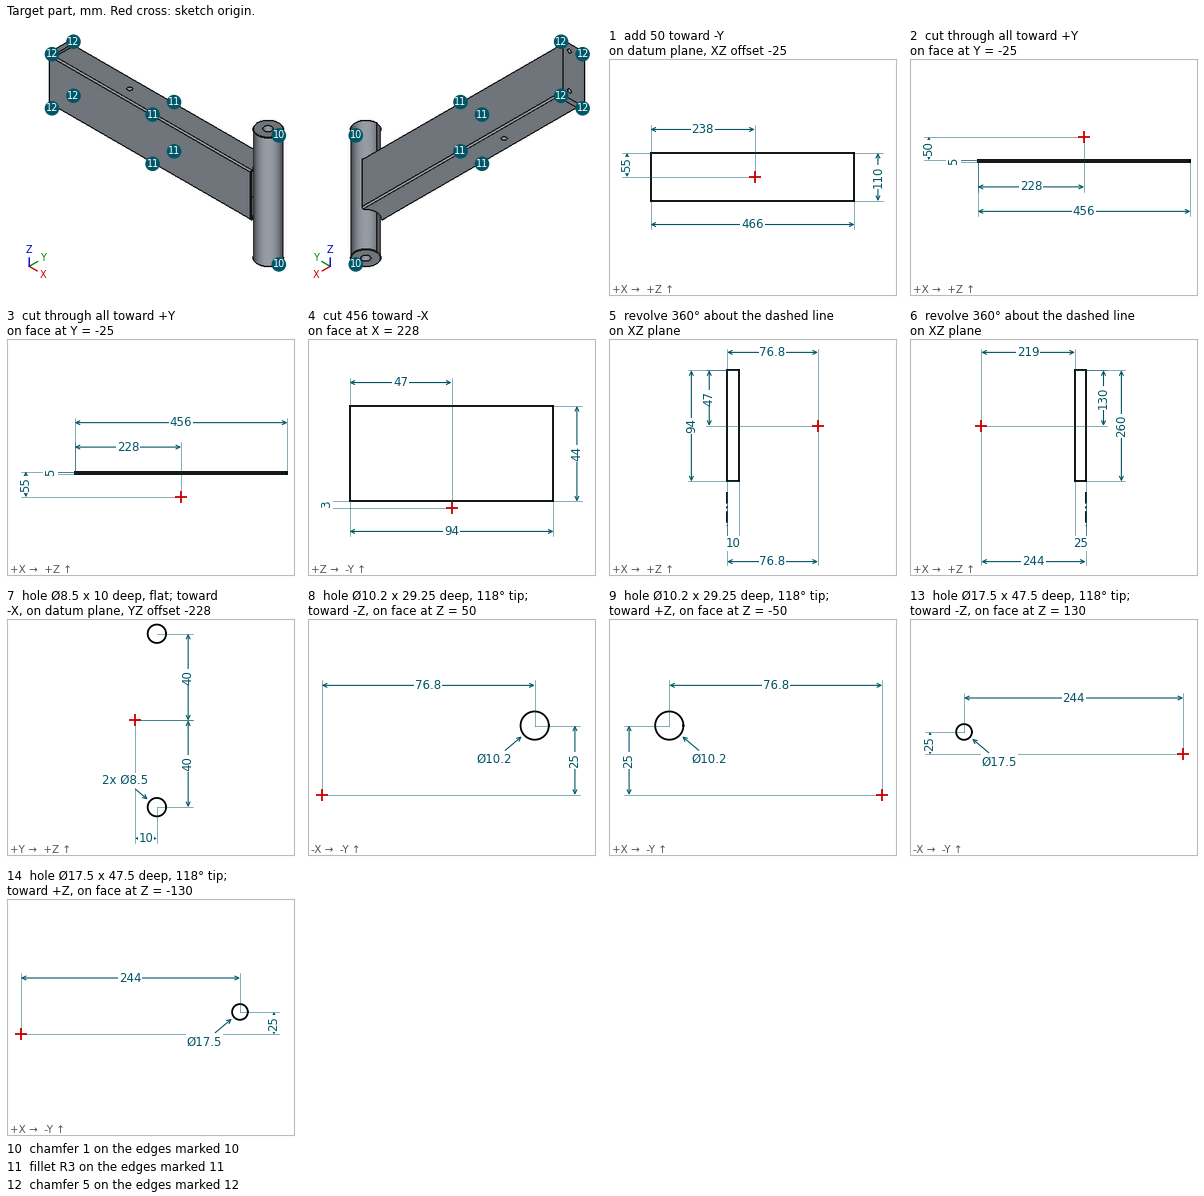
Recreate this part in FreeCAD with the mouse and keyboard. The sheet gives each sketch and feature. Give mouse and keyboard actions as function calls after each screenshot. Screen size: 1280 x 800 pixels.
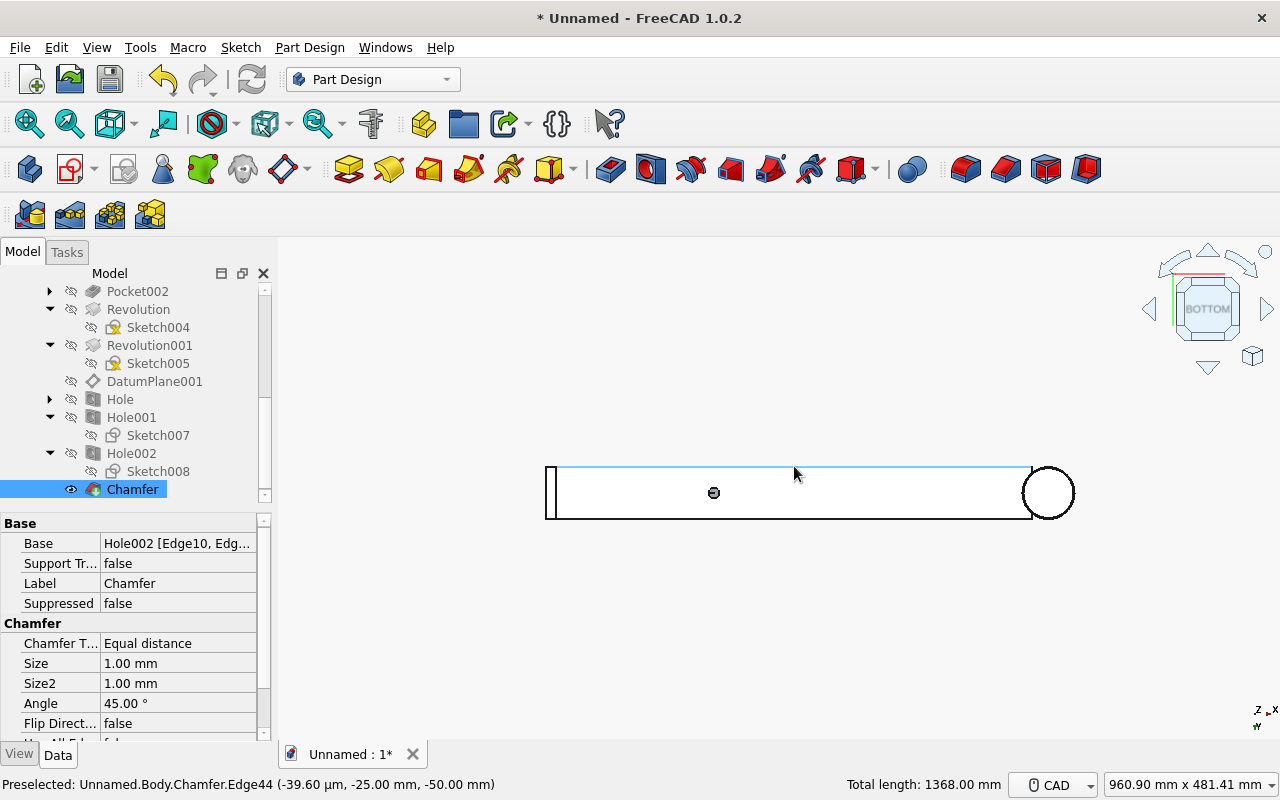
key(4)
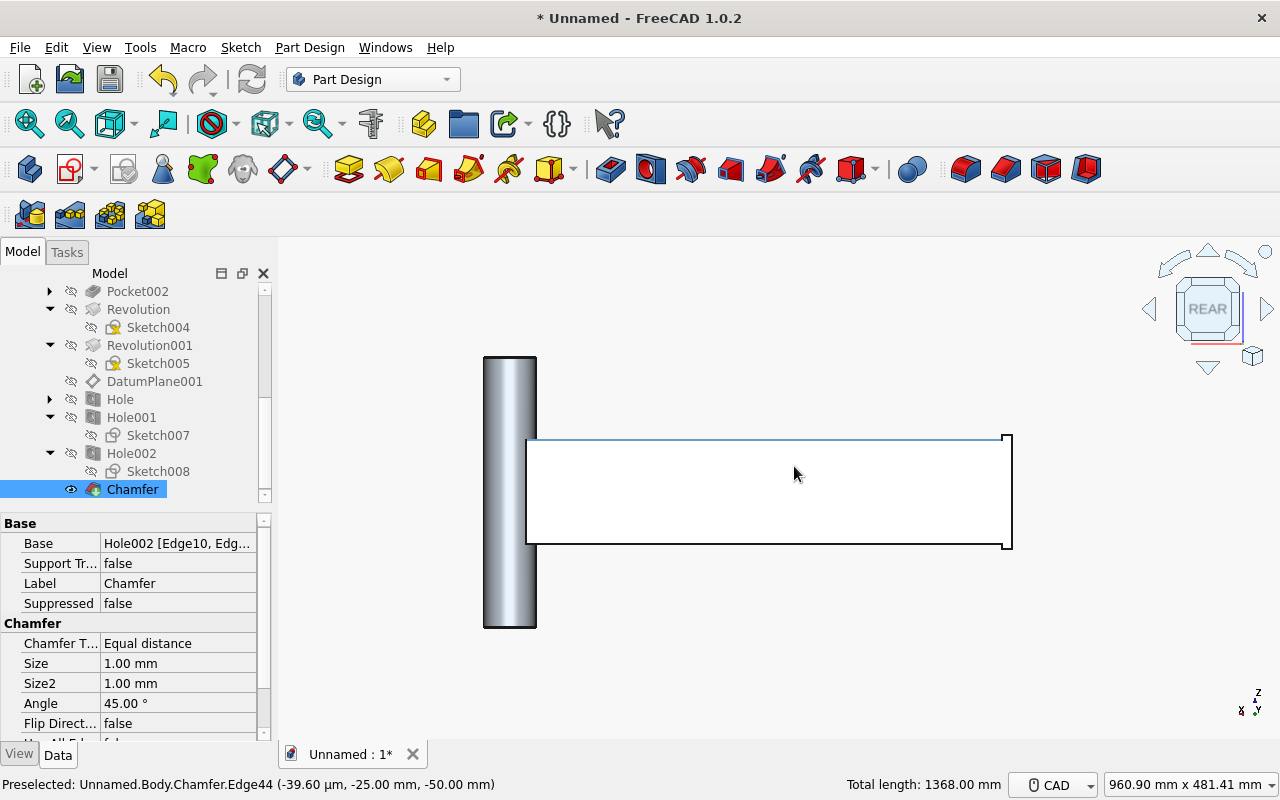
click(764, 543, ctrl)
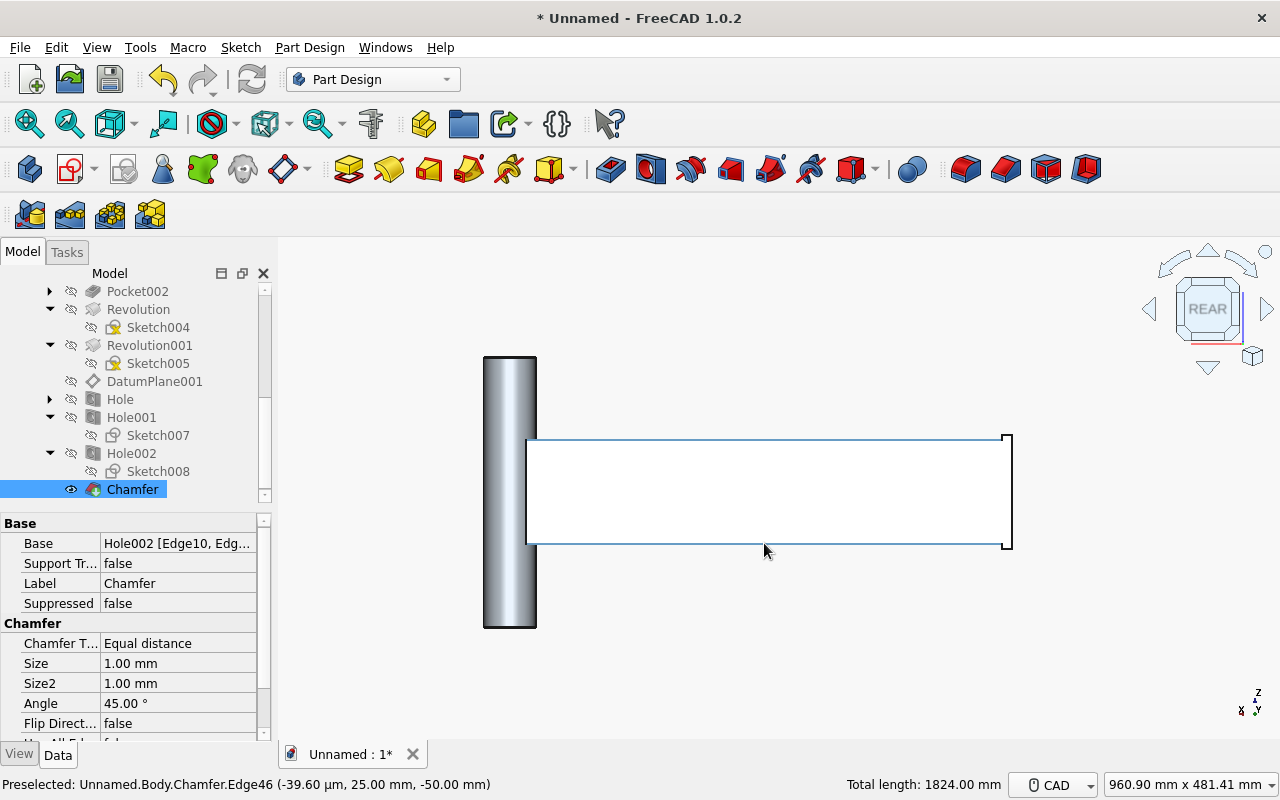
click(966, 170)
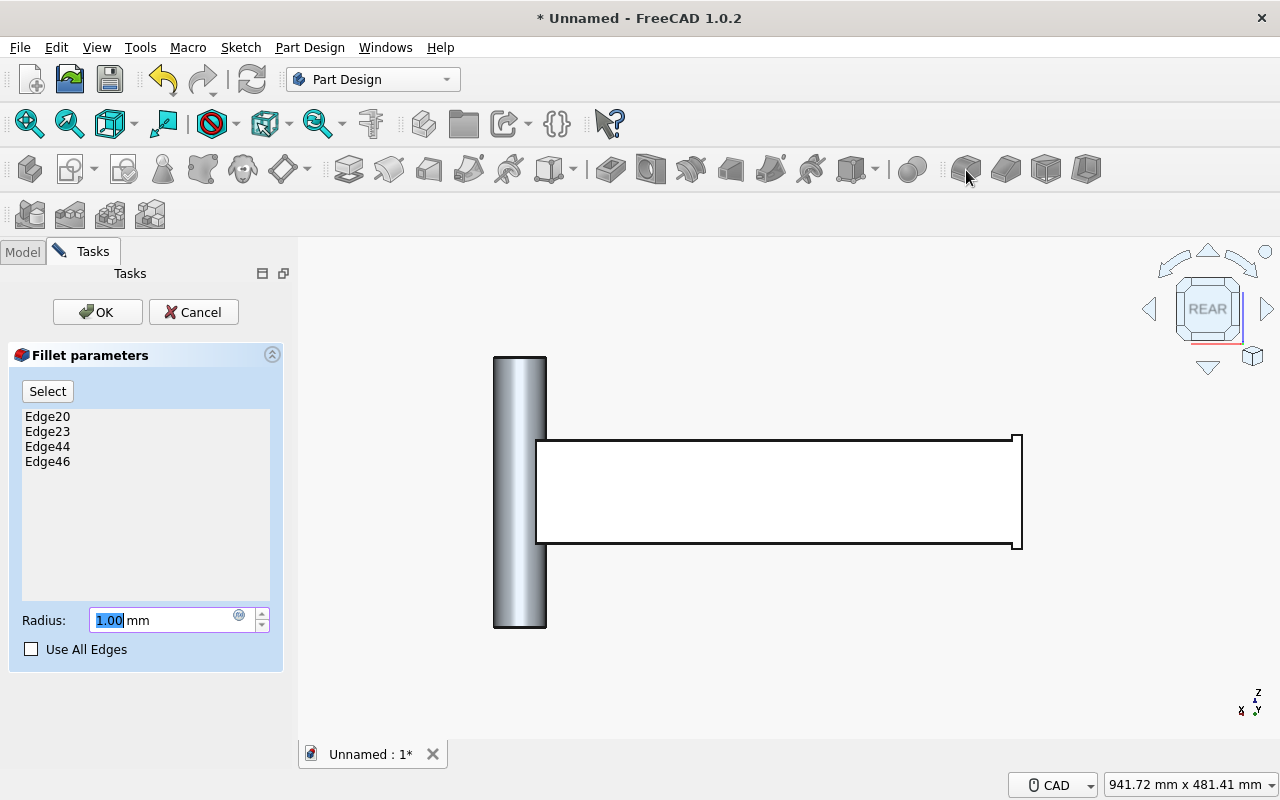
text(3)
key(Tab)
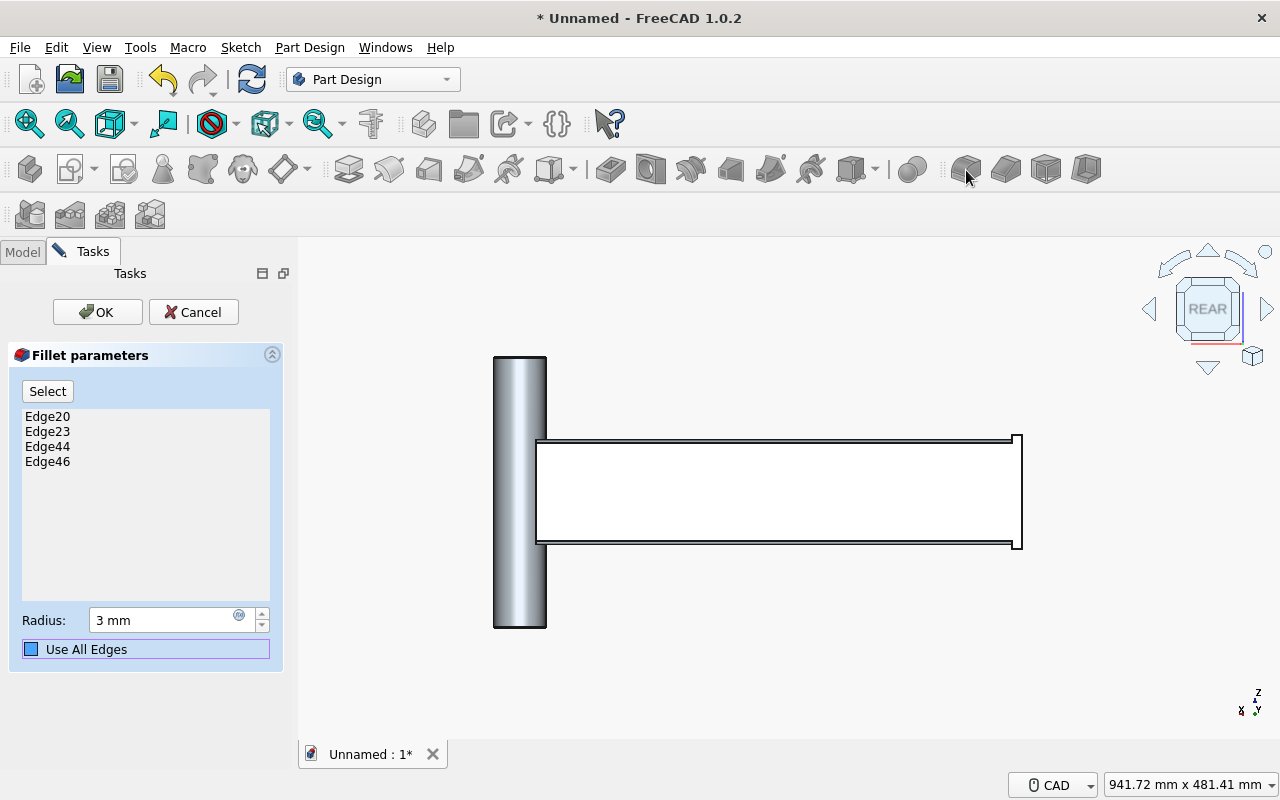
click(98, 312)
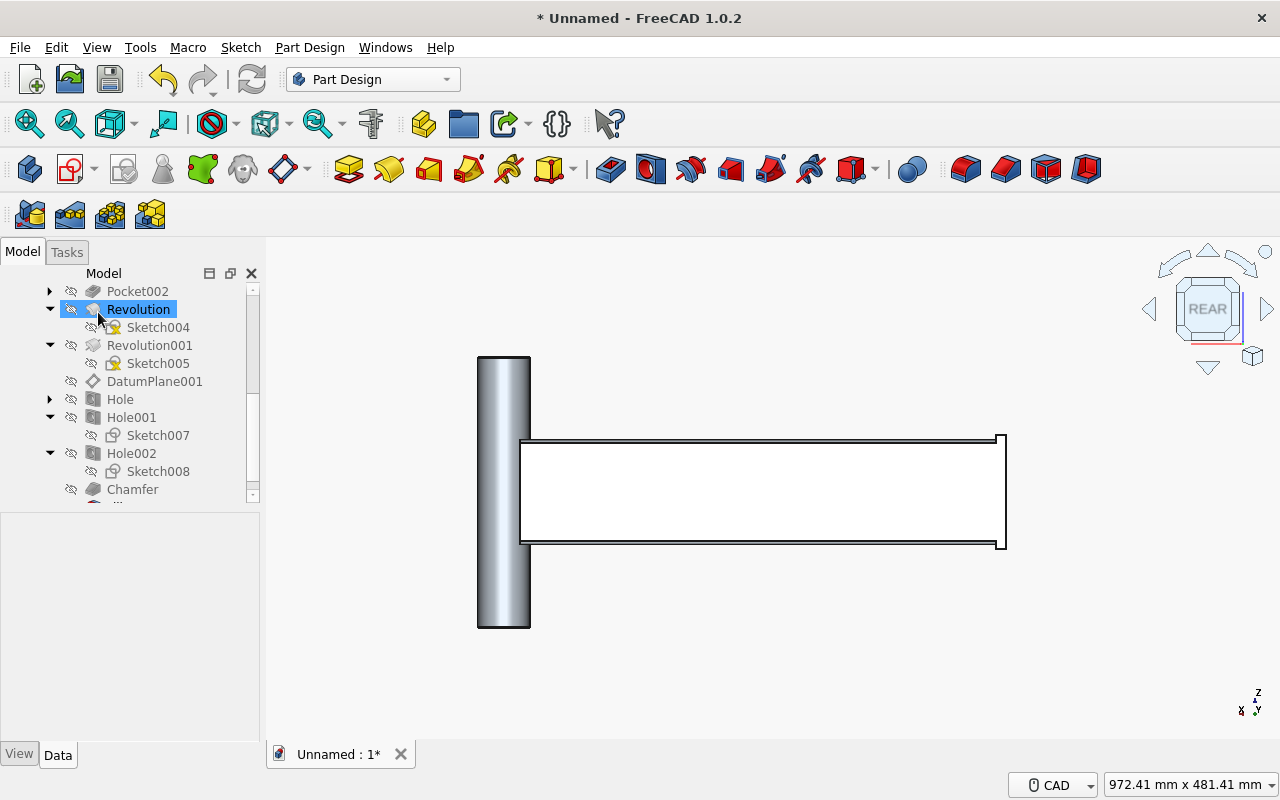
scroll(1001, 548, up, 7)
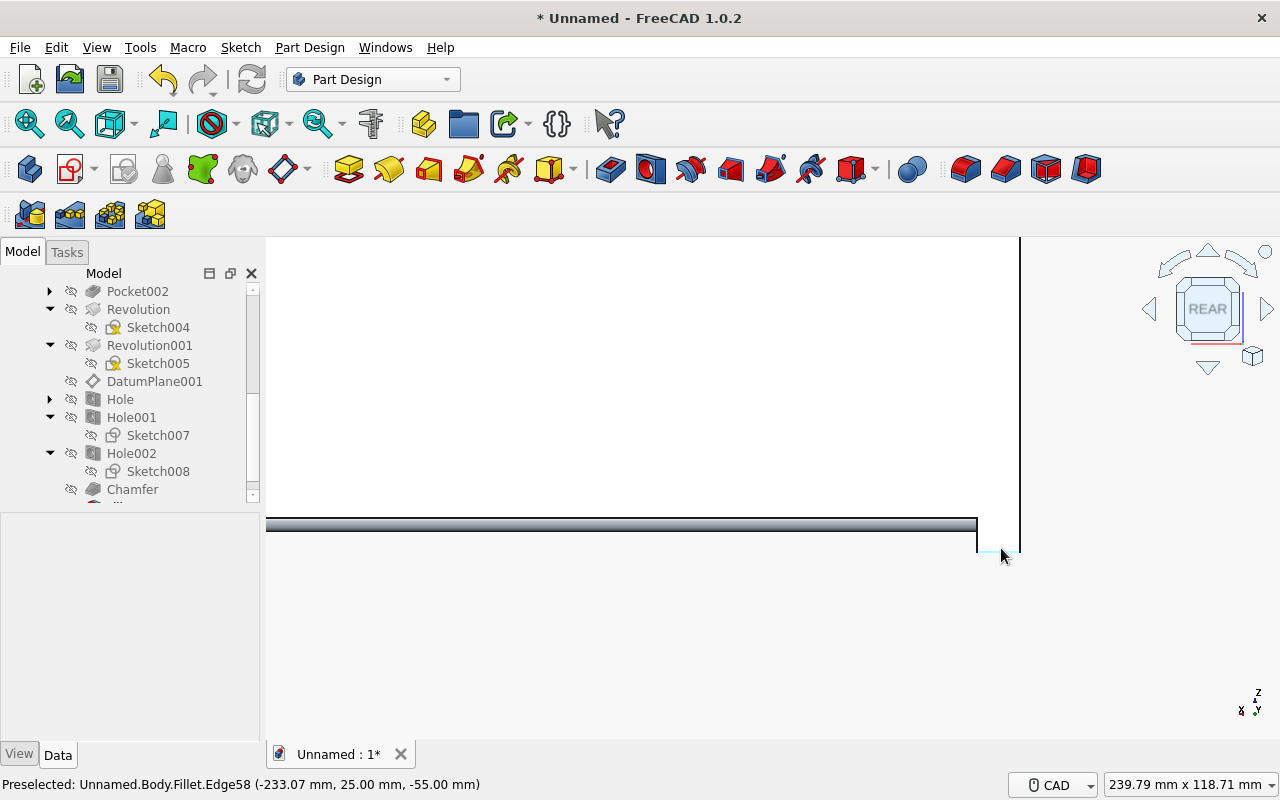
click(998, 551)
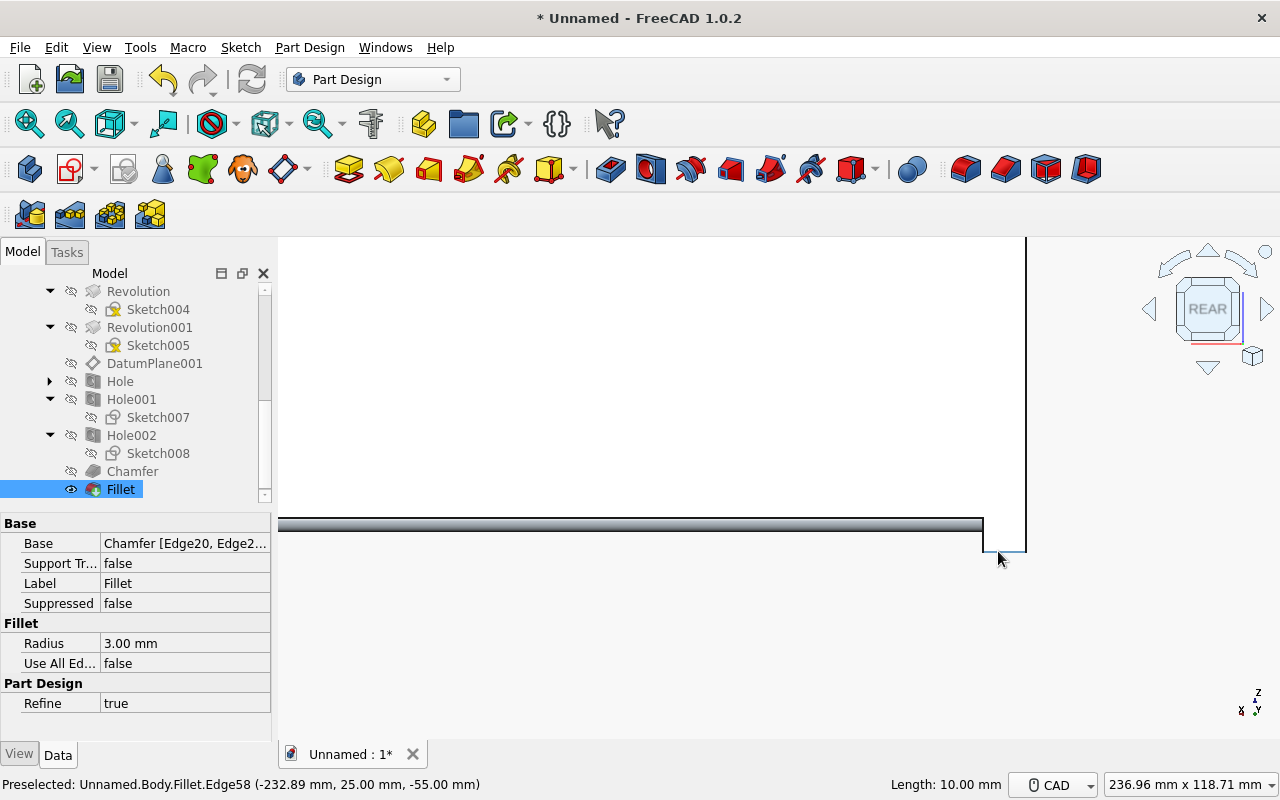
click(30, 124)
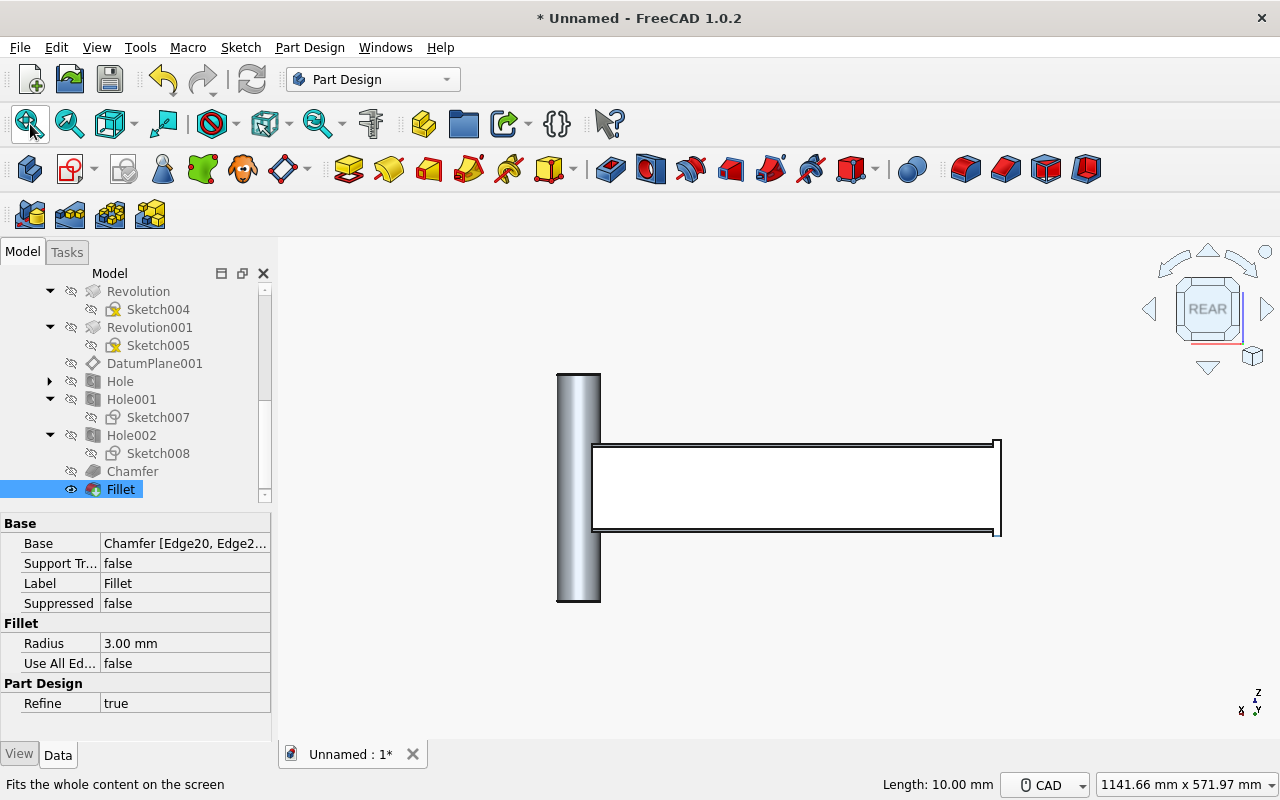
key(0)